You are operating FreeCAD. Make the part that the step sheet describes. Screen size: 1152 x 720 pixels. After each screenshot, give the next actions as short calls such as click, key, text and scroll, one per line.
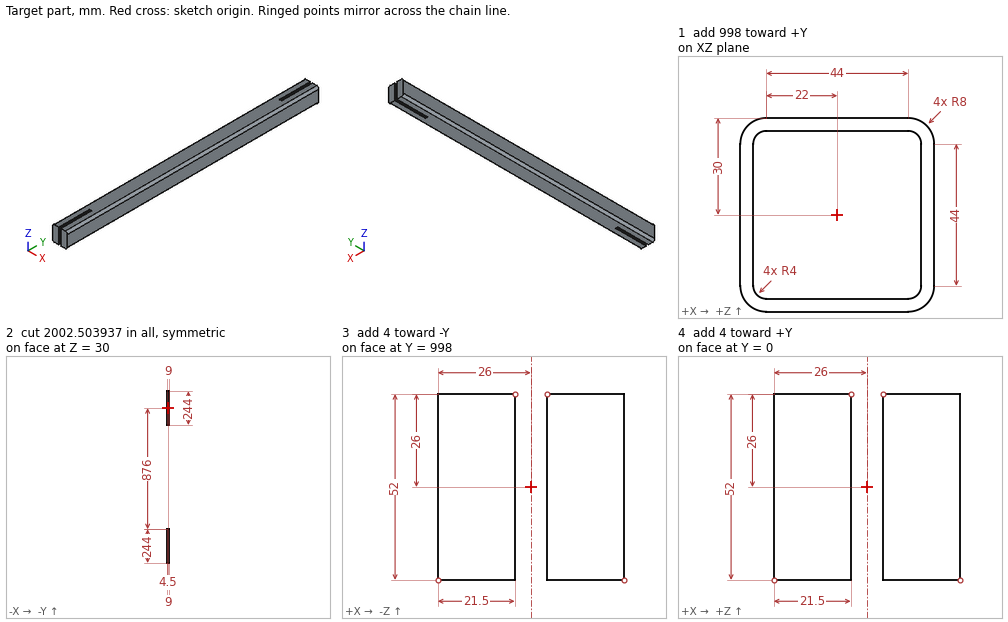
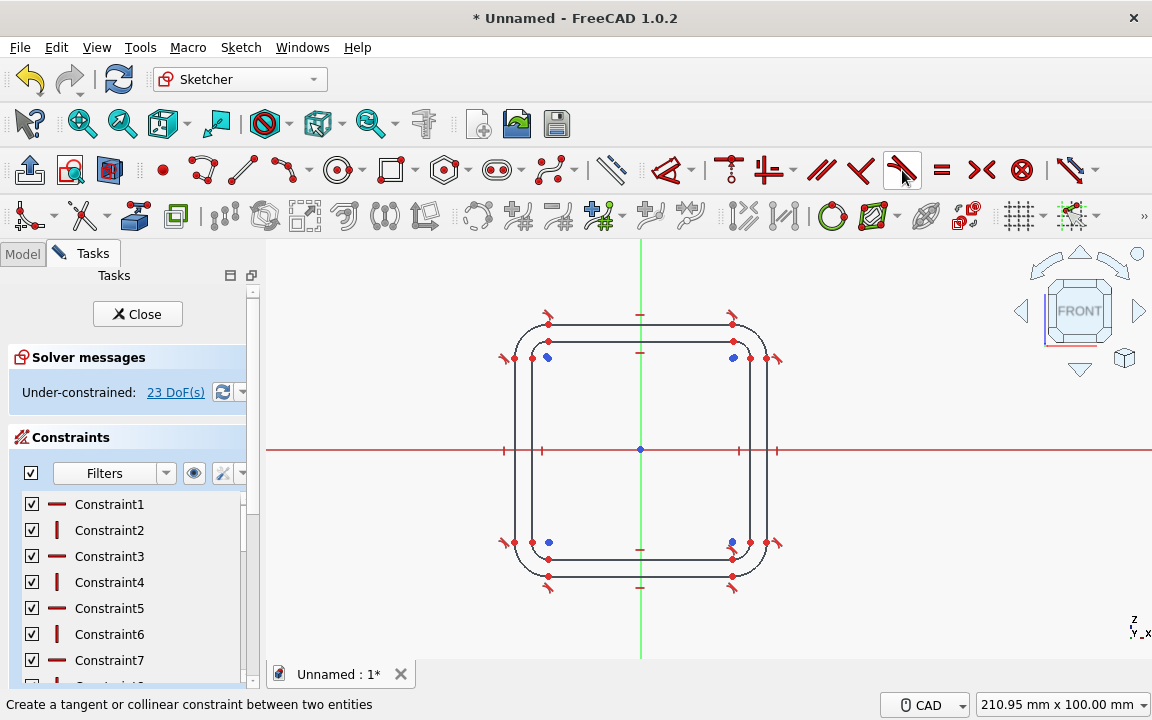
click(603, 560)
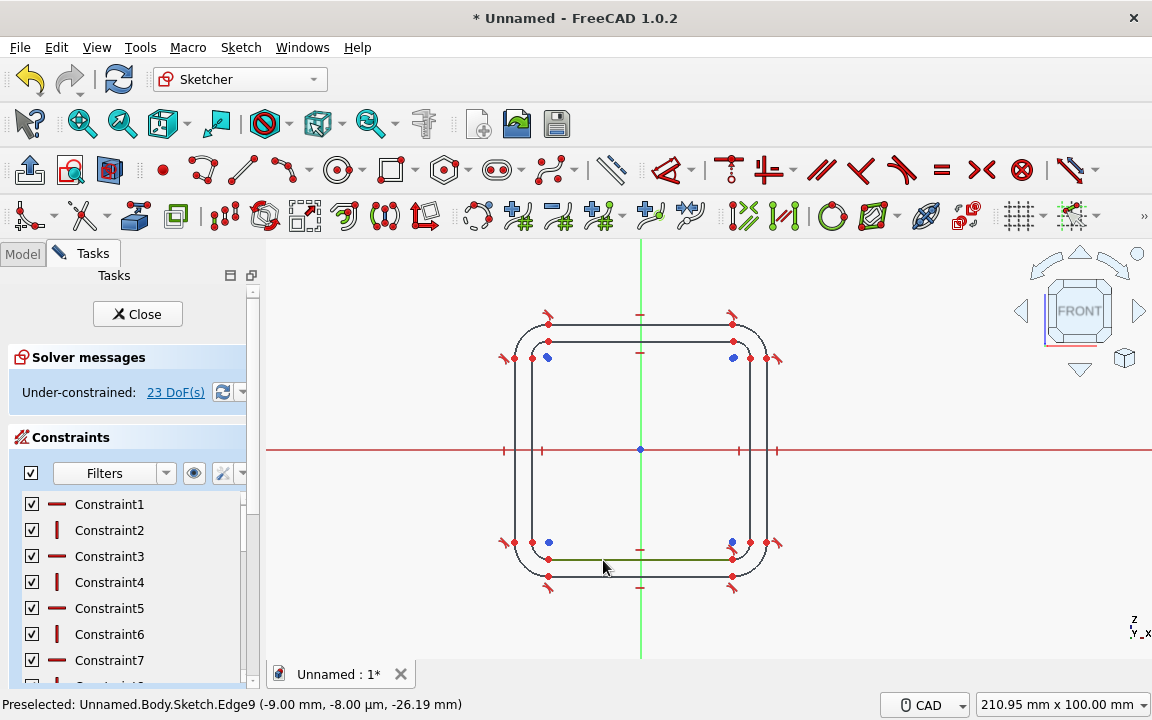
click(537, 554)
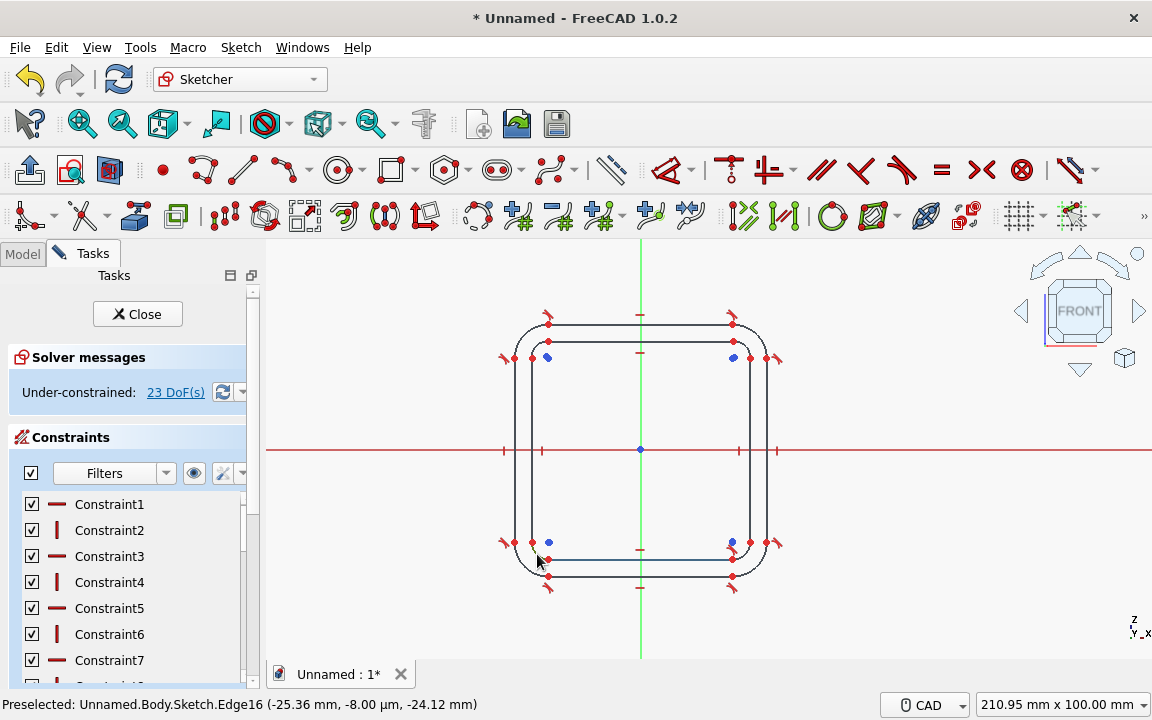
click(902, 170)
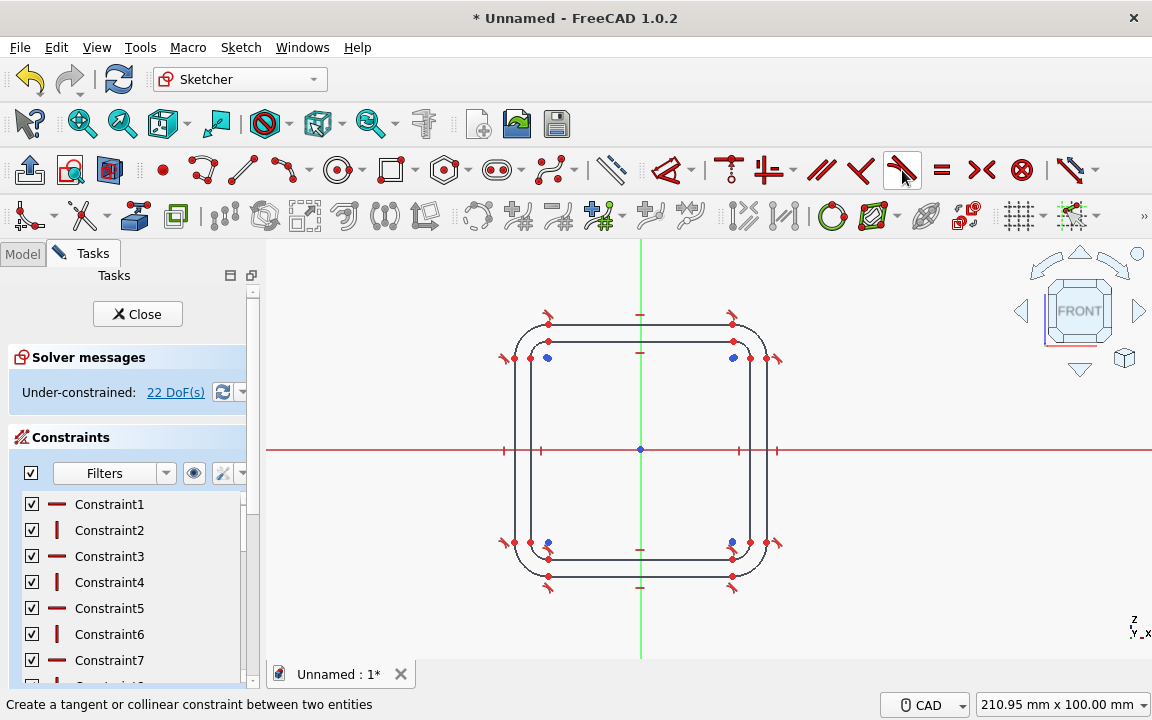
click(750, 488)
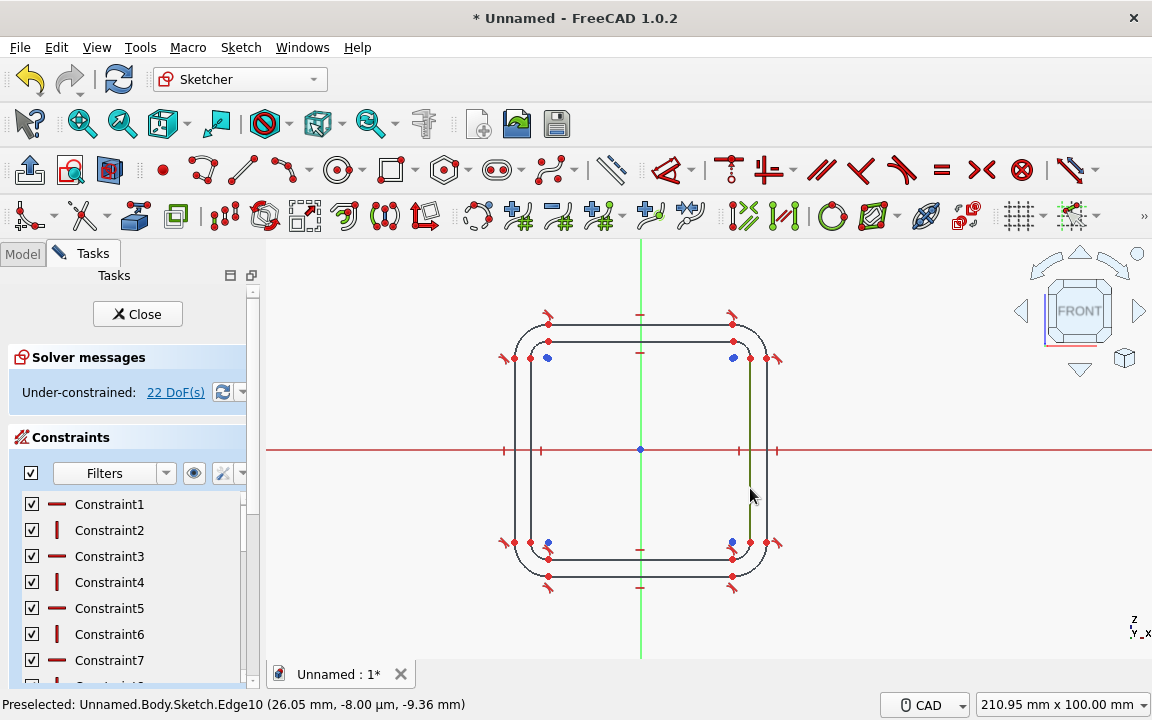
click(745, 555)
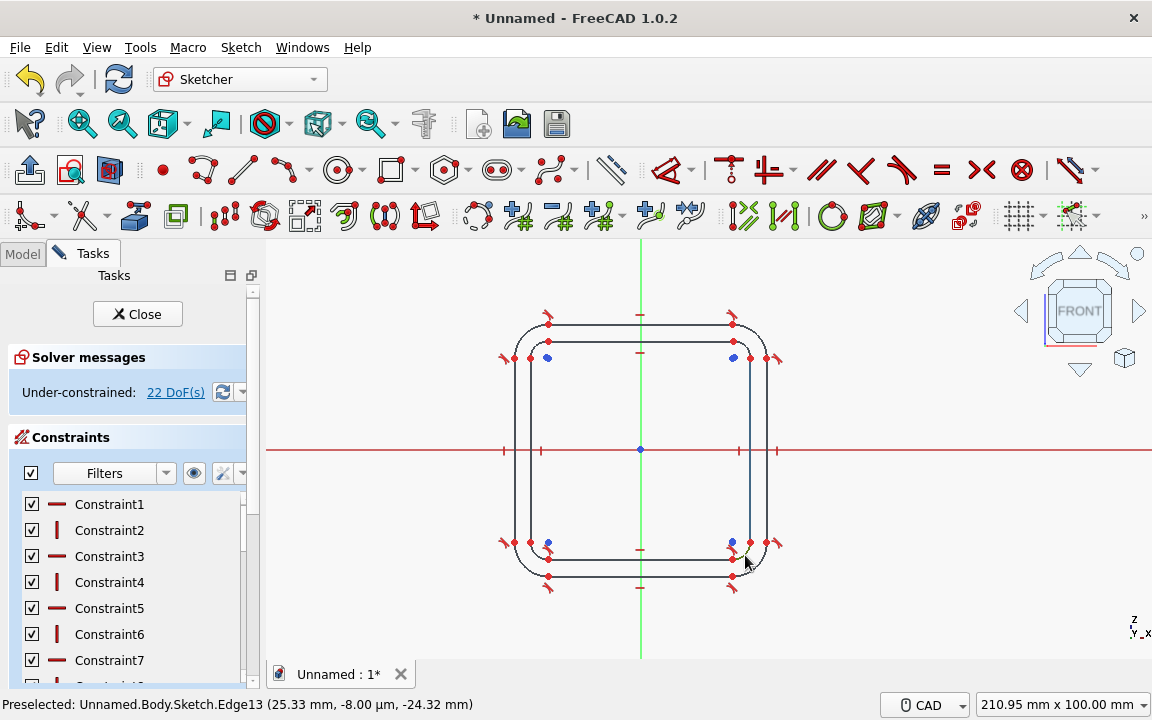
click(902, 170)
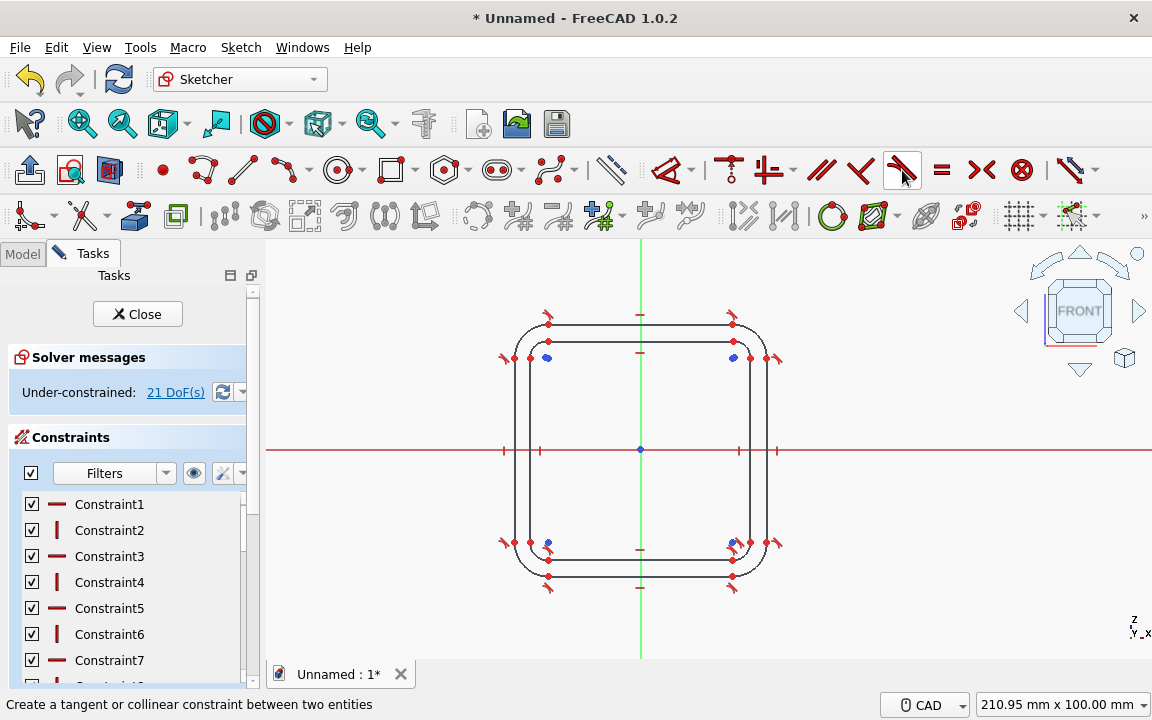
click(750, 487)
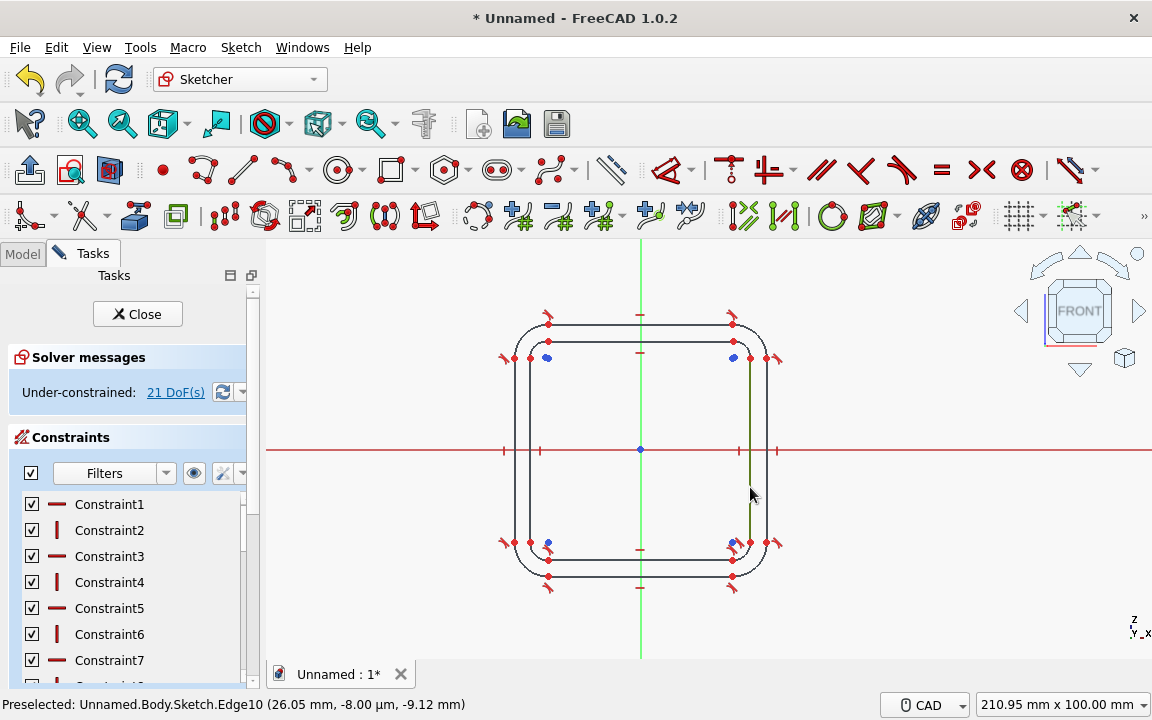
click(746, 346)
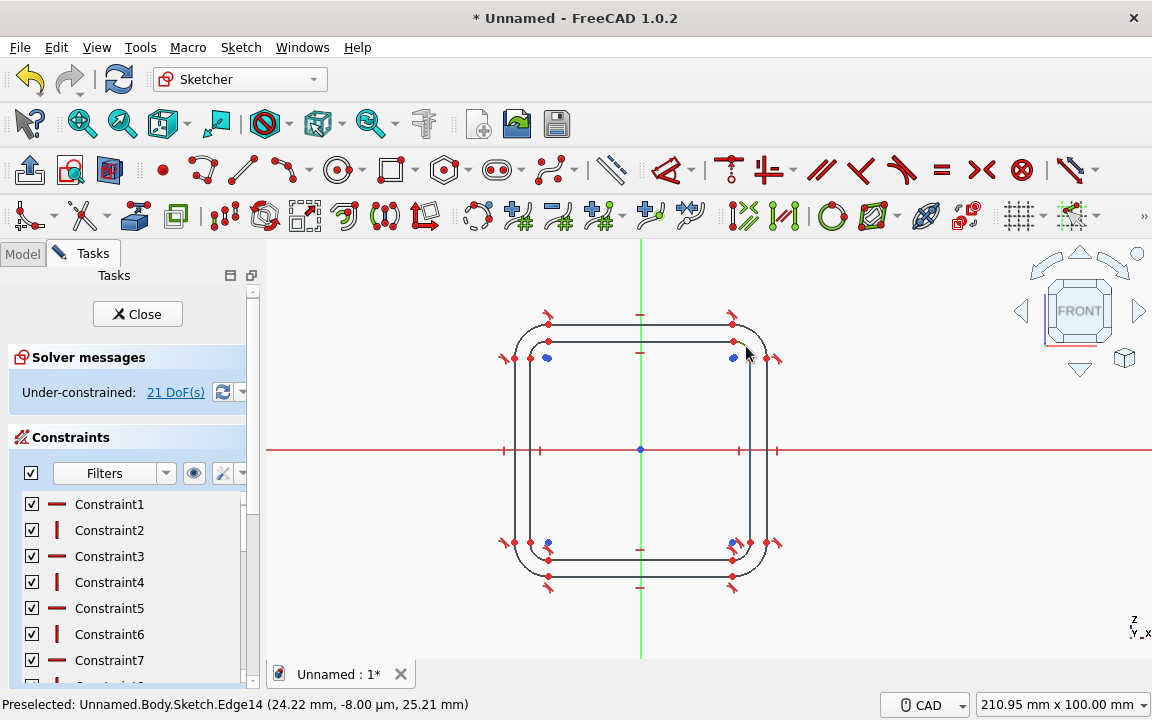
click(902, 170)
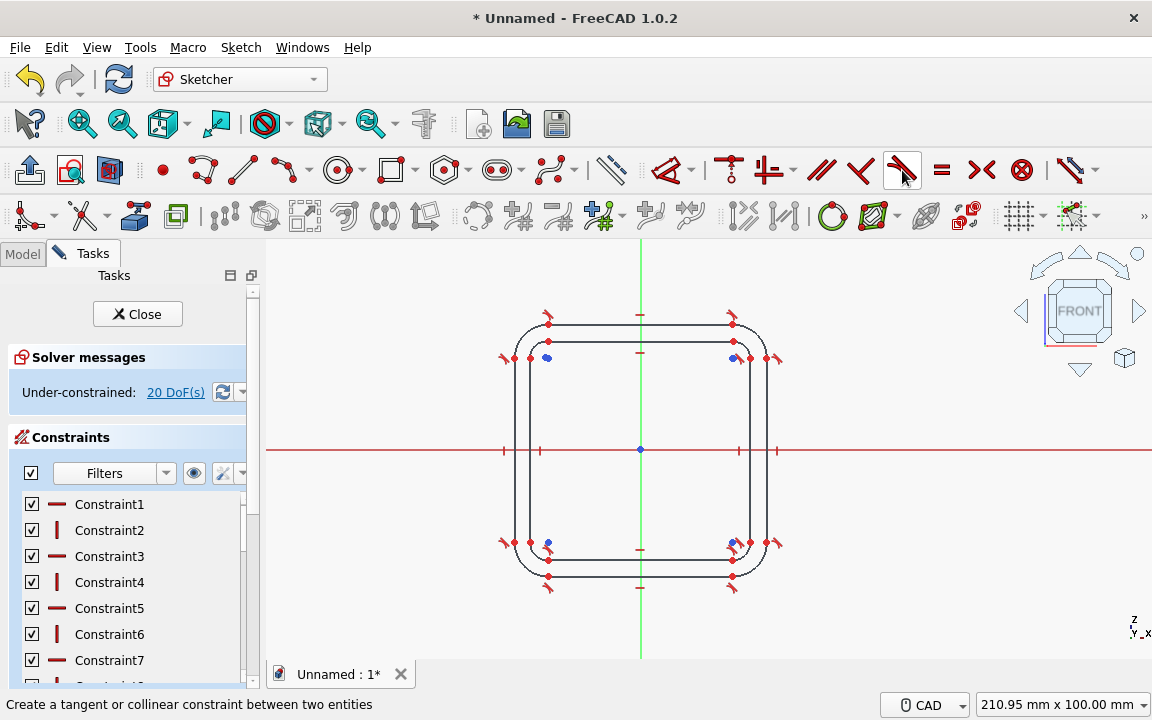
click(677, 342)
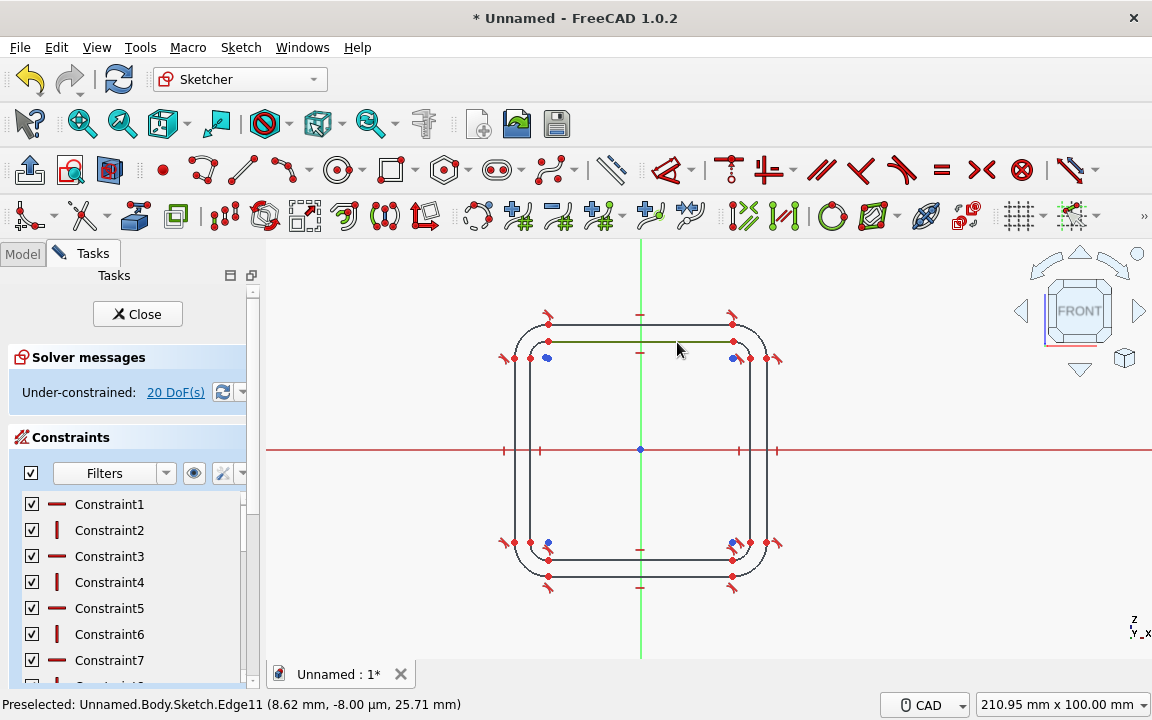
click(745, 347)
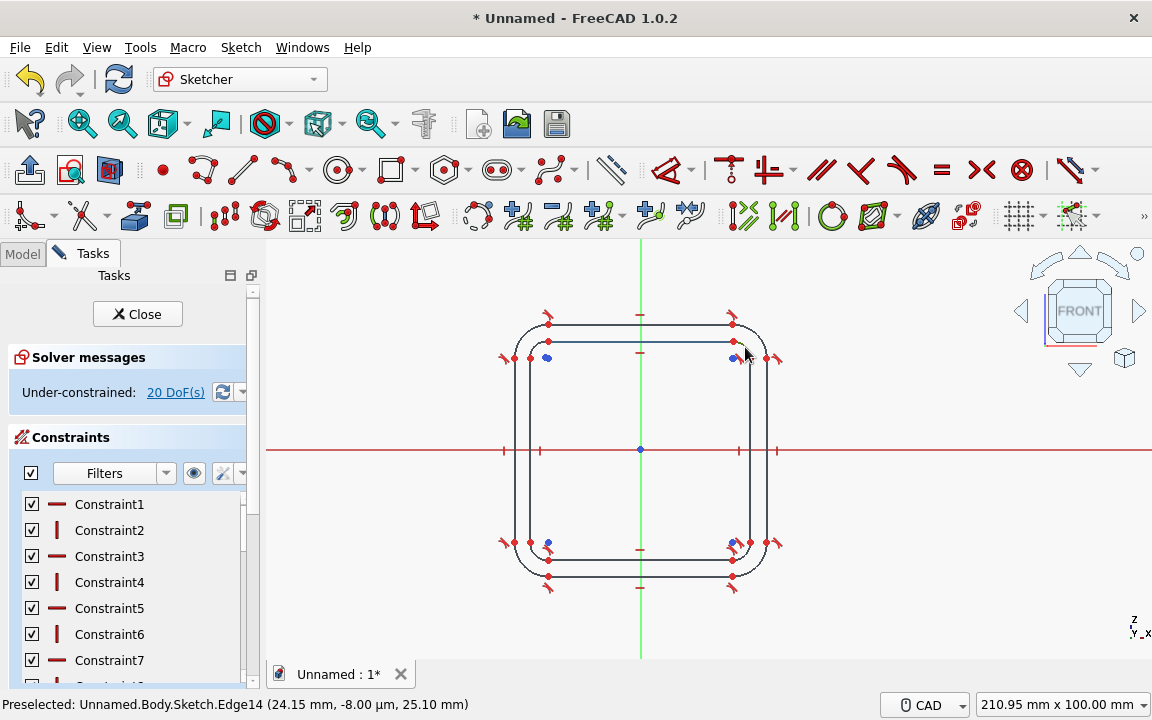
click(902, 170)